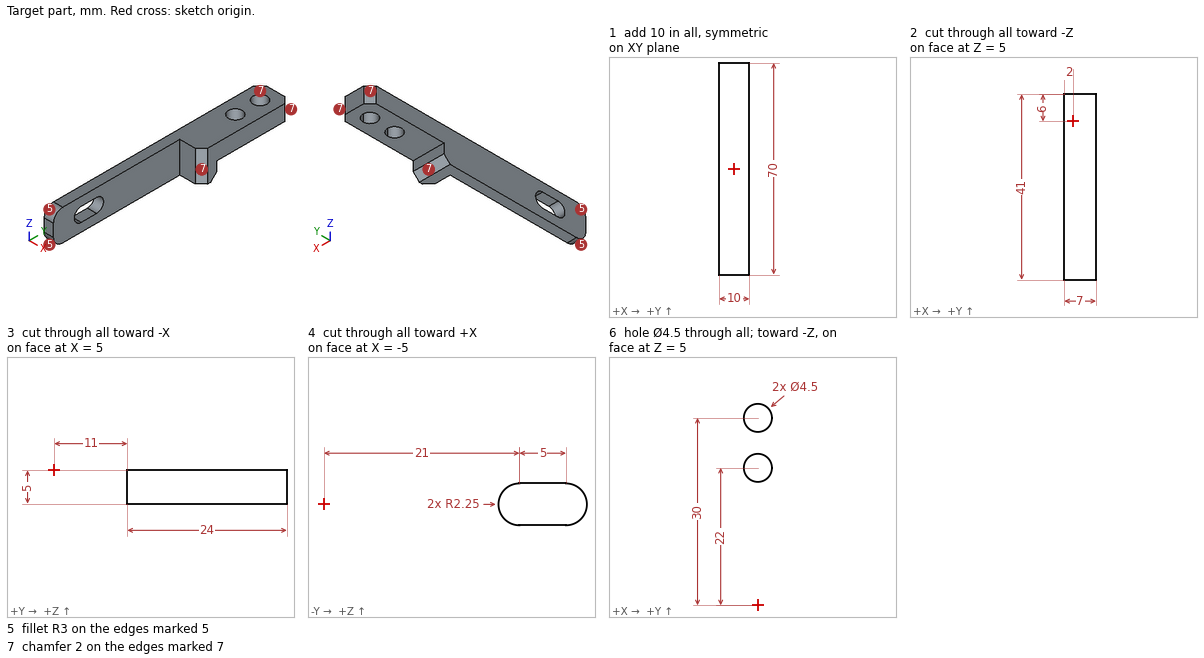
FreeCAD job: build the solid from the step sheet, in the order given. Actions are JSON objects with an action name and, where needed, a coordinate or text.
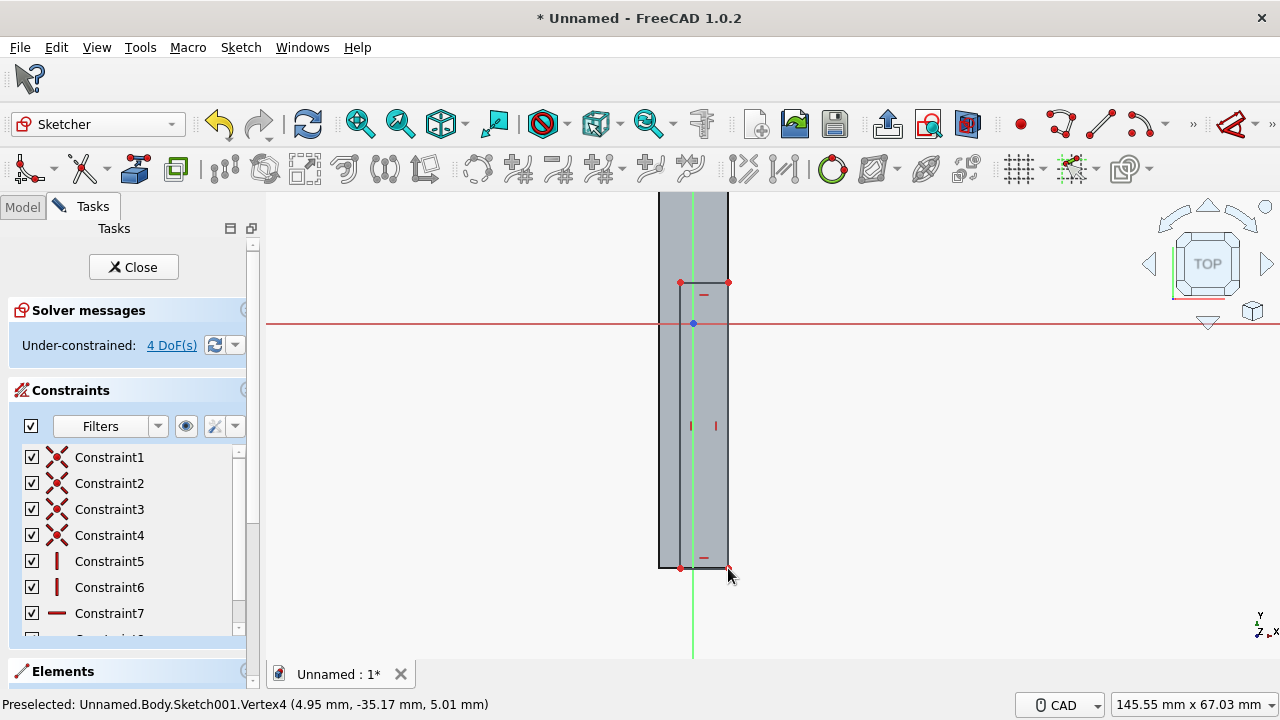
{"action": "key", "text": "d"}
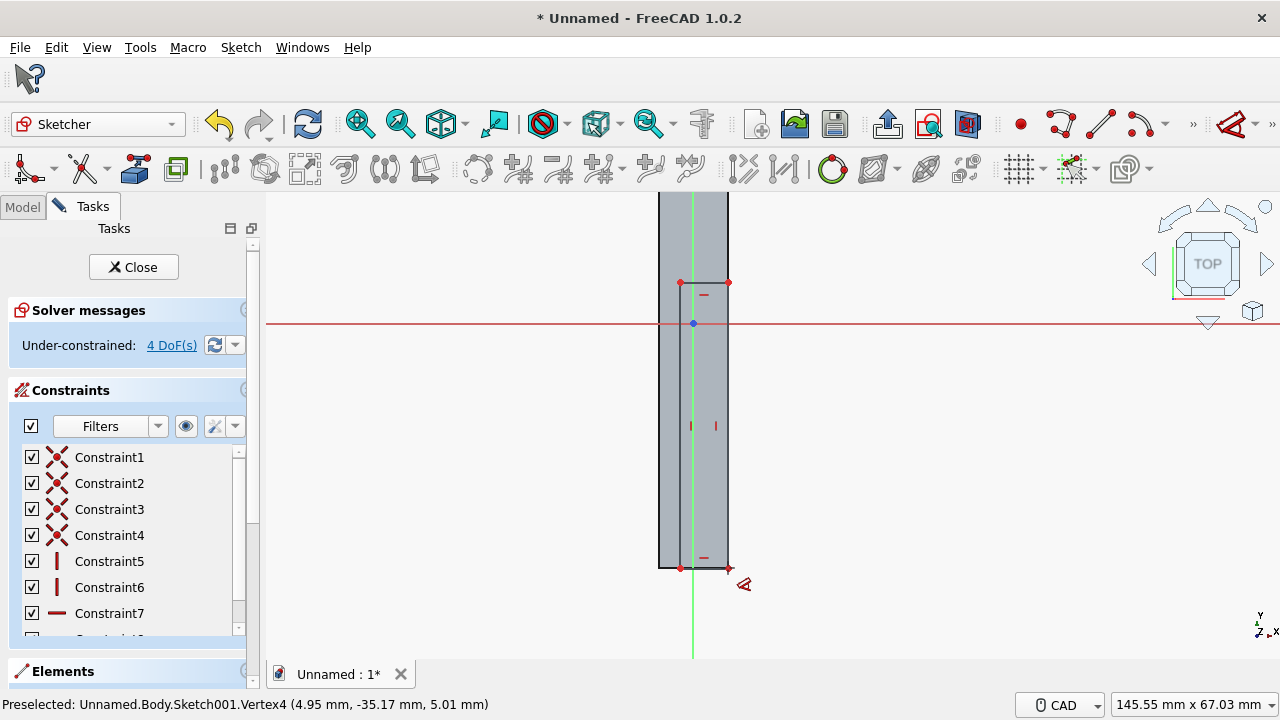
{"action": "left_click", "coordinate": [694, 569]}
{"action": "left_click", "coordinate": [715, 603]}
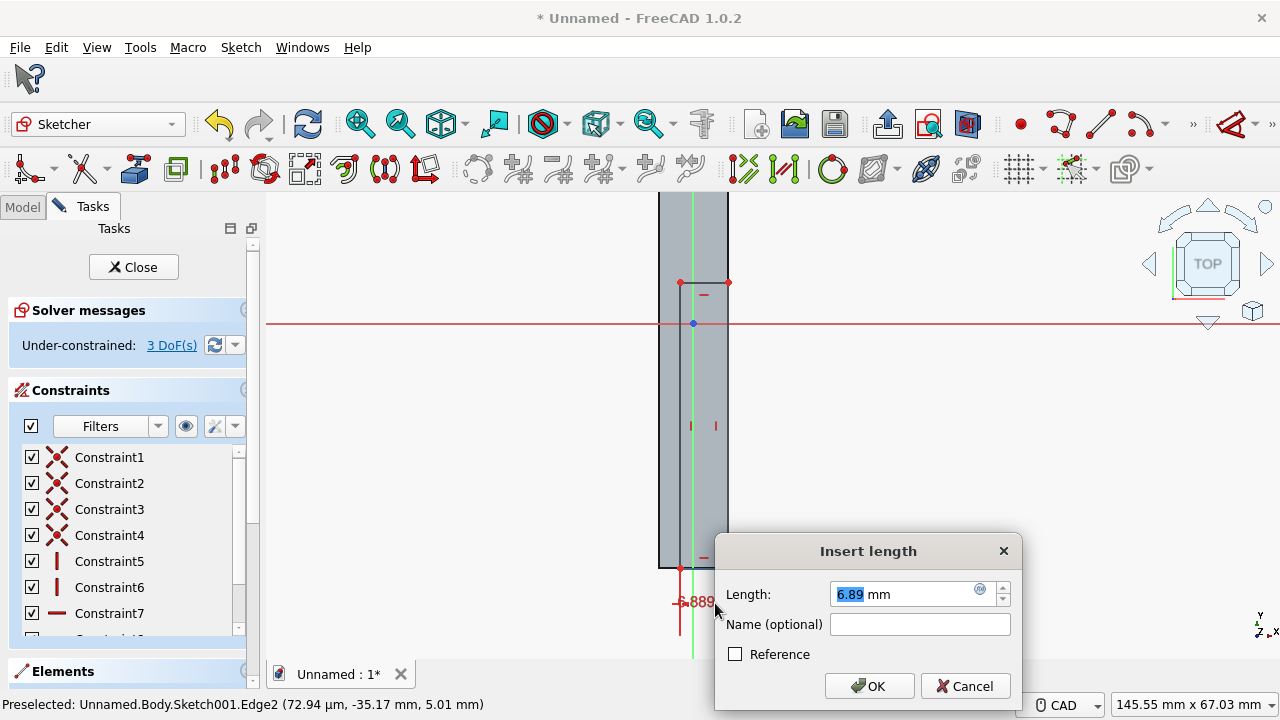
{"action": "type", "text": "7"}
{"action": "key", "text": "Return"}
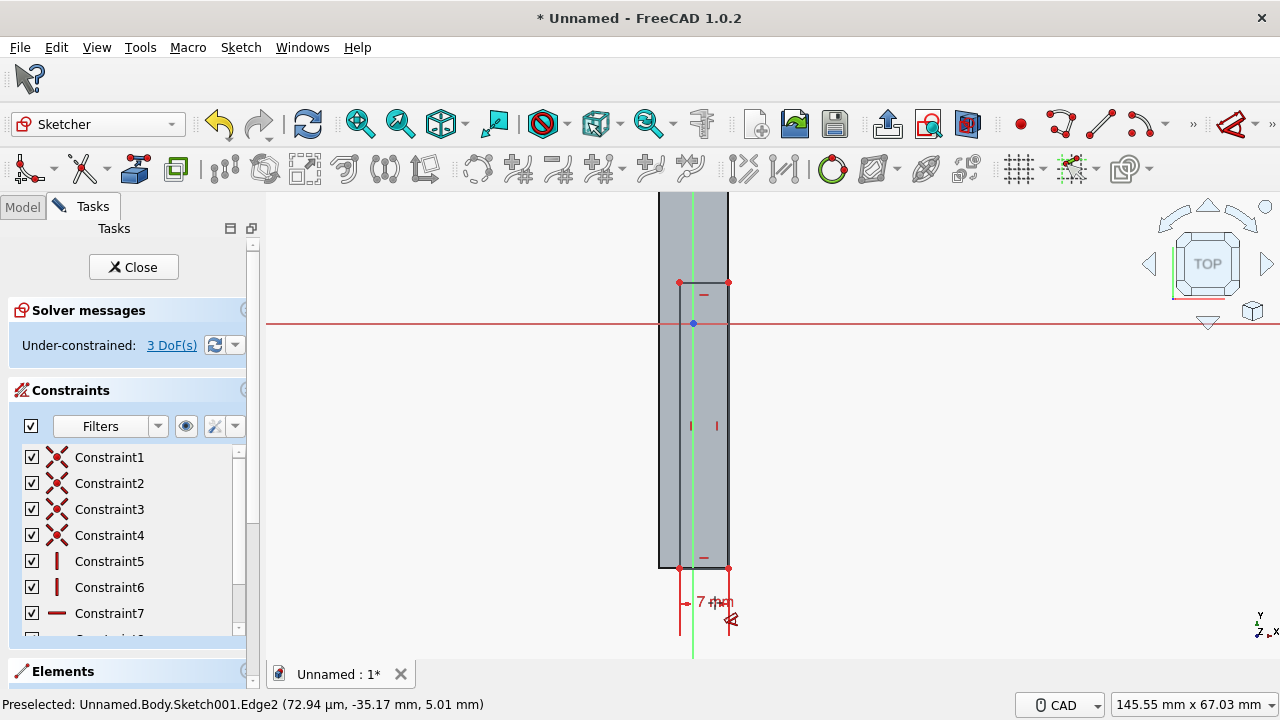
{"action": "left_click", "coordinate": [680, 369]}
{"action": "left_click", "coordinate": [646, 426]}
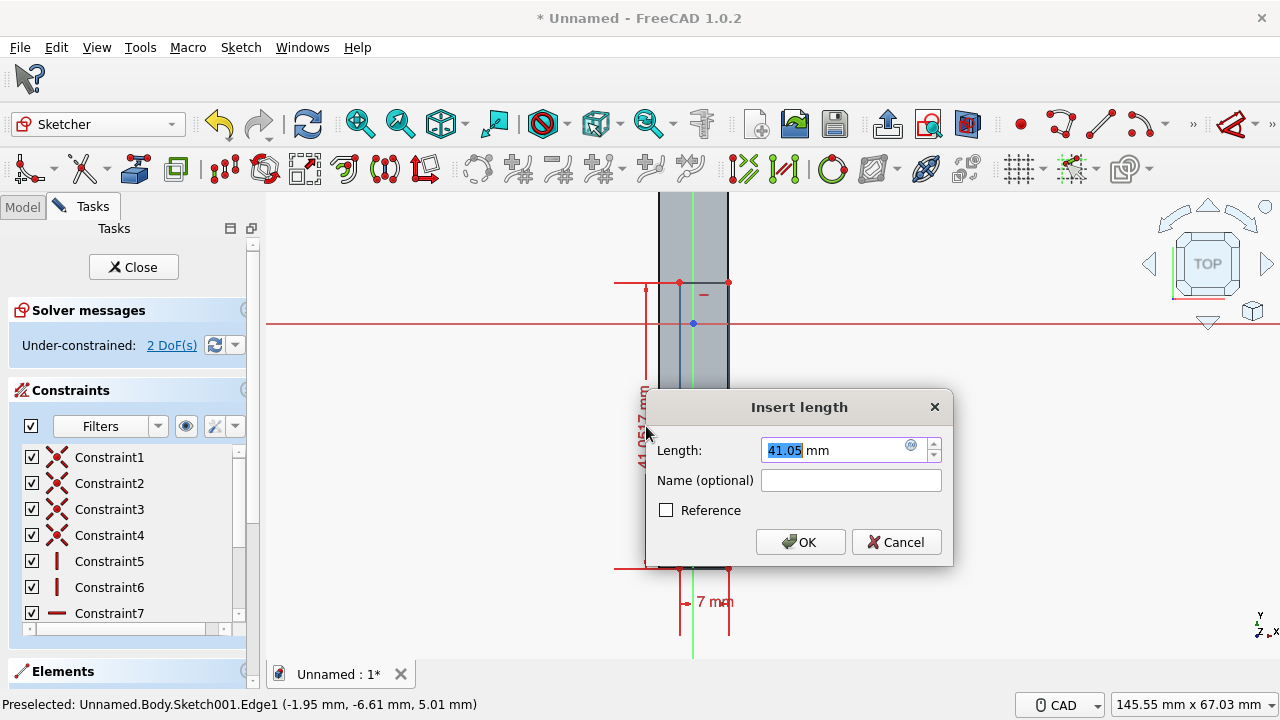
{"action": "type", "text": "41"}
{"action": "key", "text": "Return"}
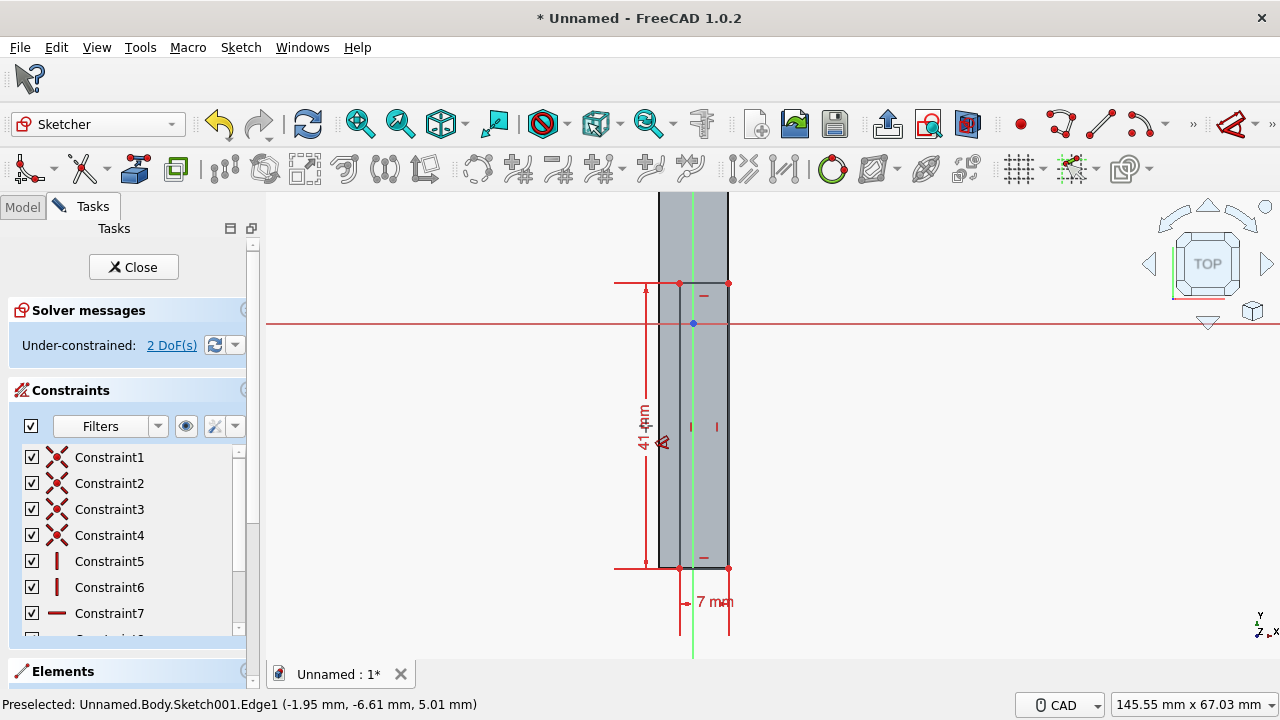
{"action": "scroll", "coordinate": [680, 283], "scroll_direction": "up", "scroll_amount": 6}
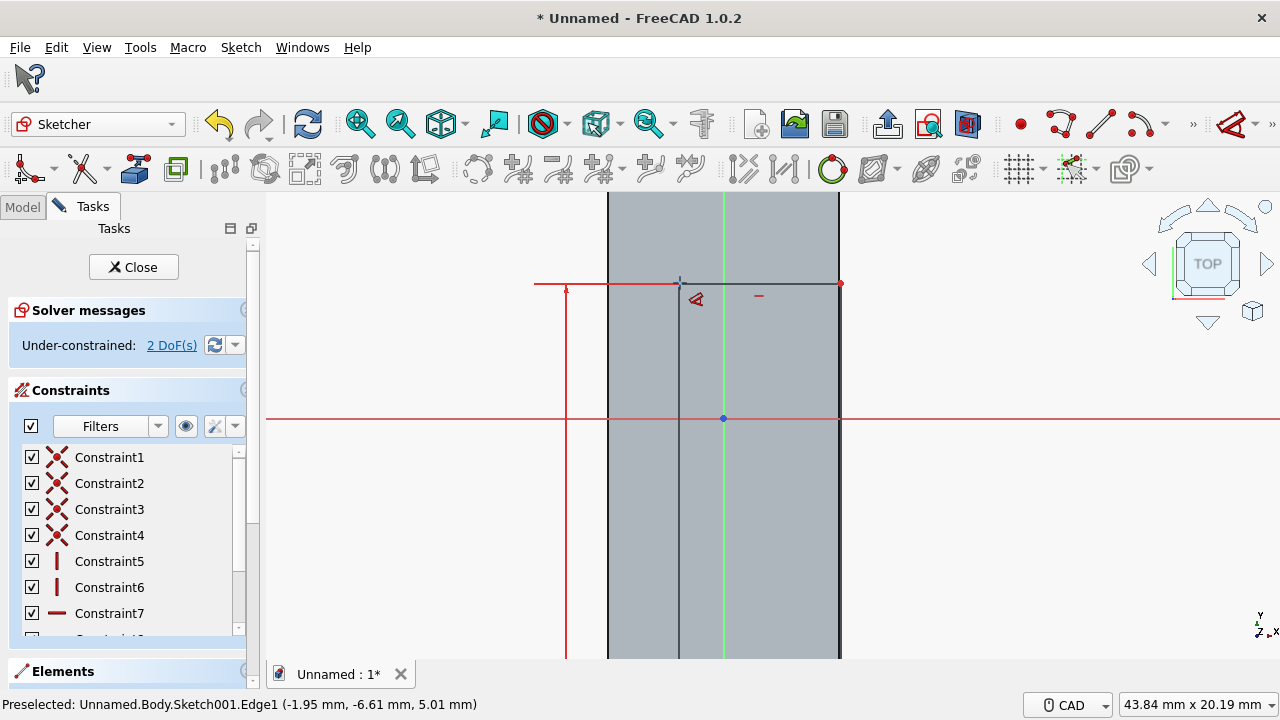
{"action": "left_click", "coordinate": [679, 284]}
{"action": "left_click", "coordinate": [701, 250]}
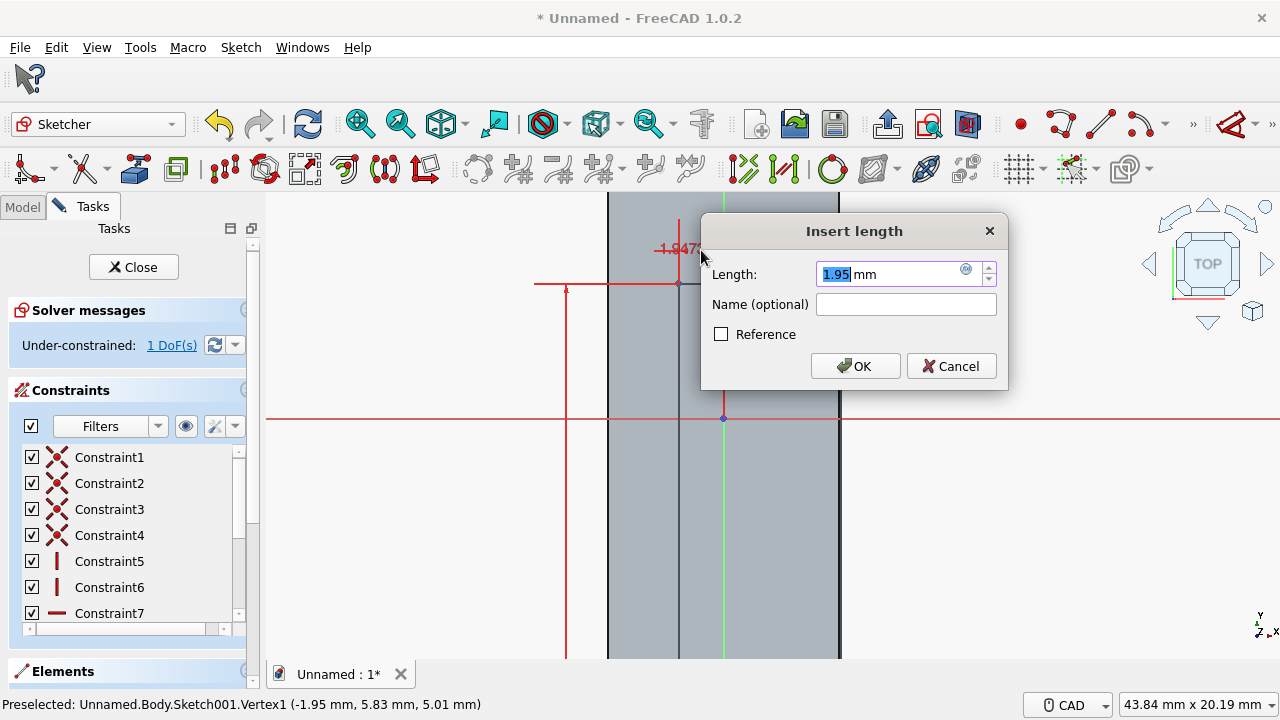
{"action": "type", "text": "2"}
{"action": "key", "text": "Return"}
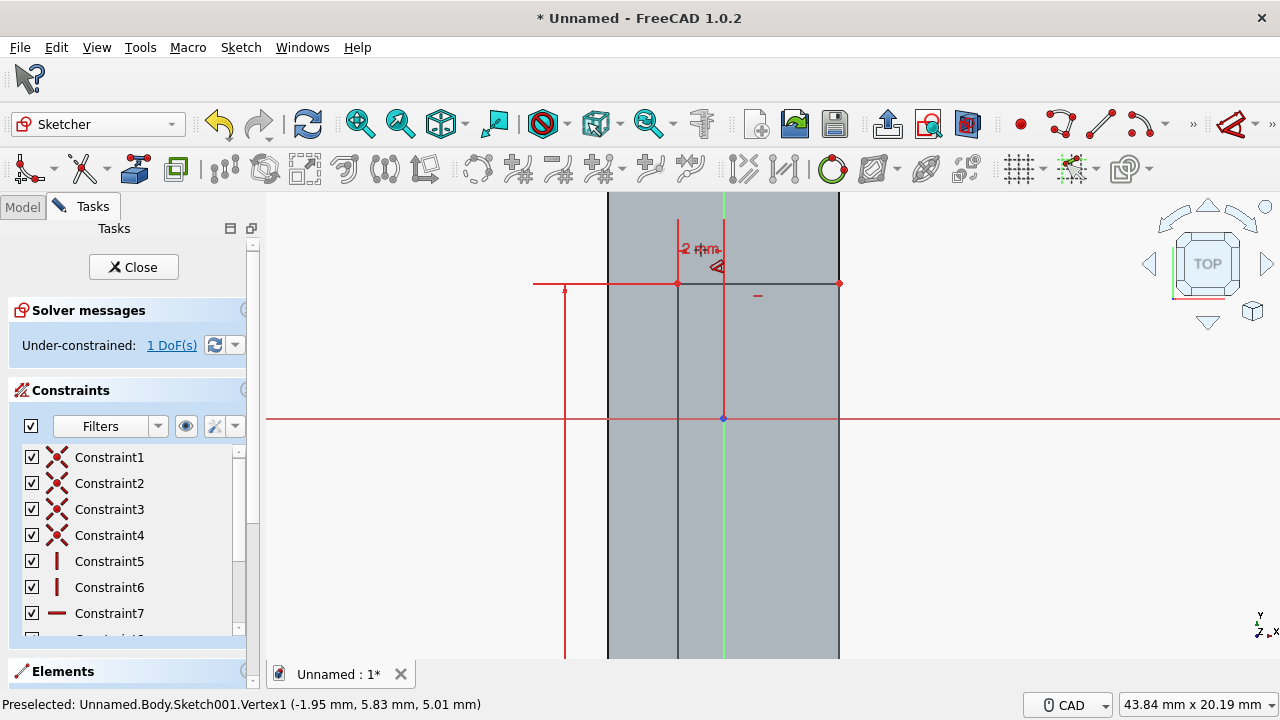
{"action": "left_click", "coordinate": [678, 284]}
{"action": "left_click", "coordinate": [644, 351]}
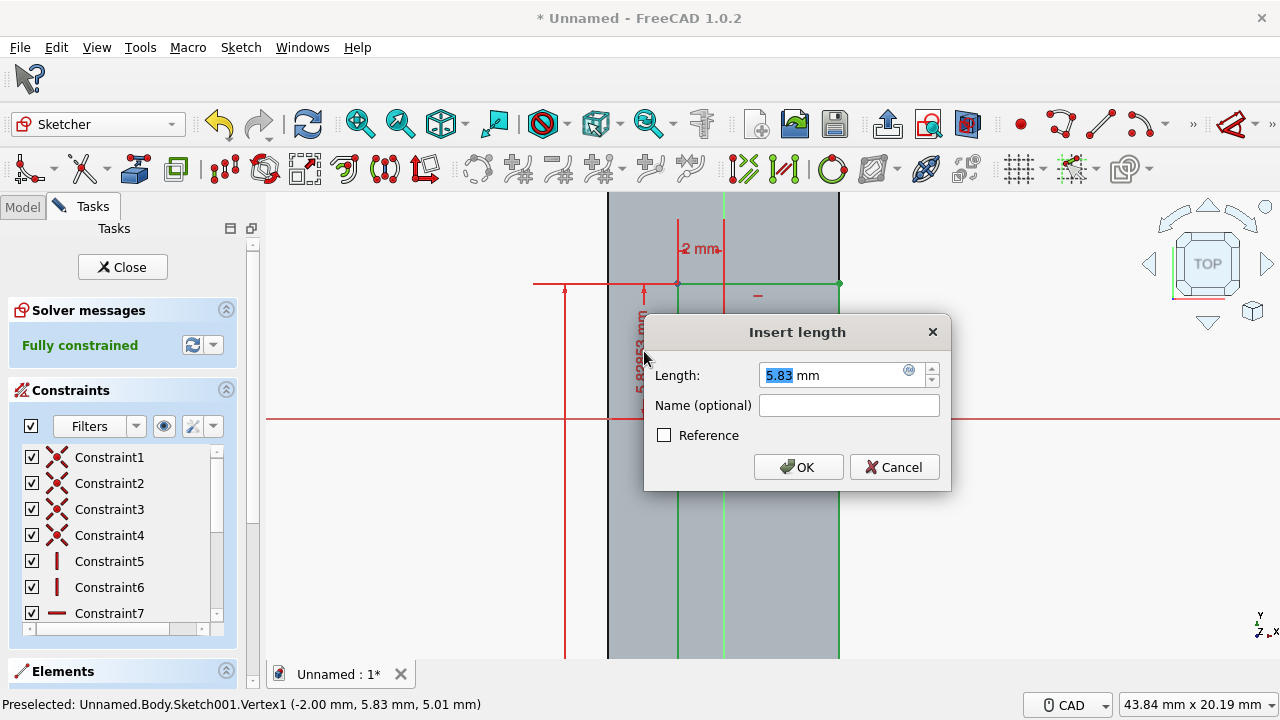
{"action": "type", "text": "6"}
{"action": "key", "text": "Return"}
{"action": "key", "text": "Escape"}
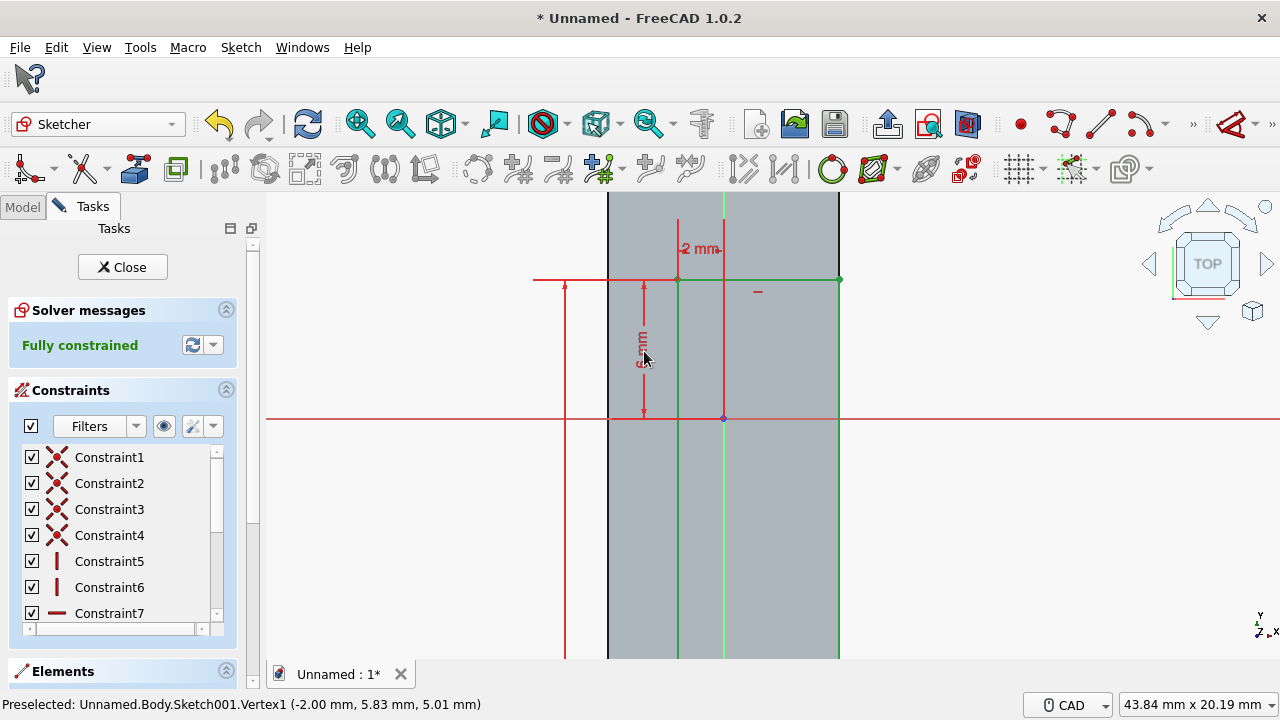
{"action": "left_click", "coordinate": [123, 267]}